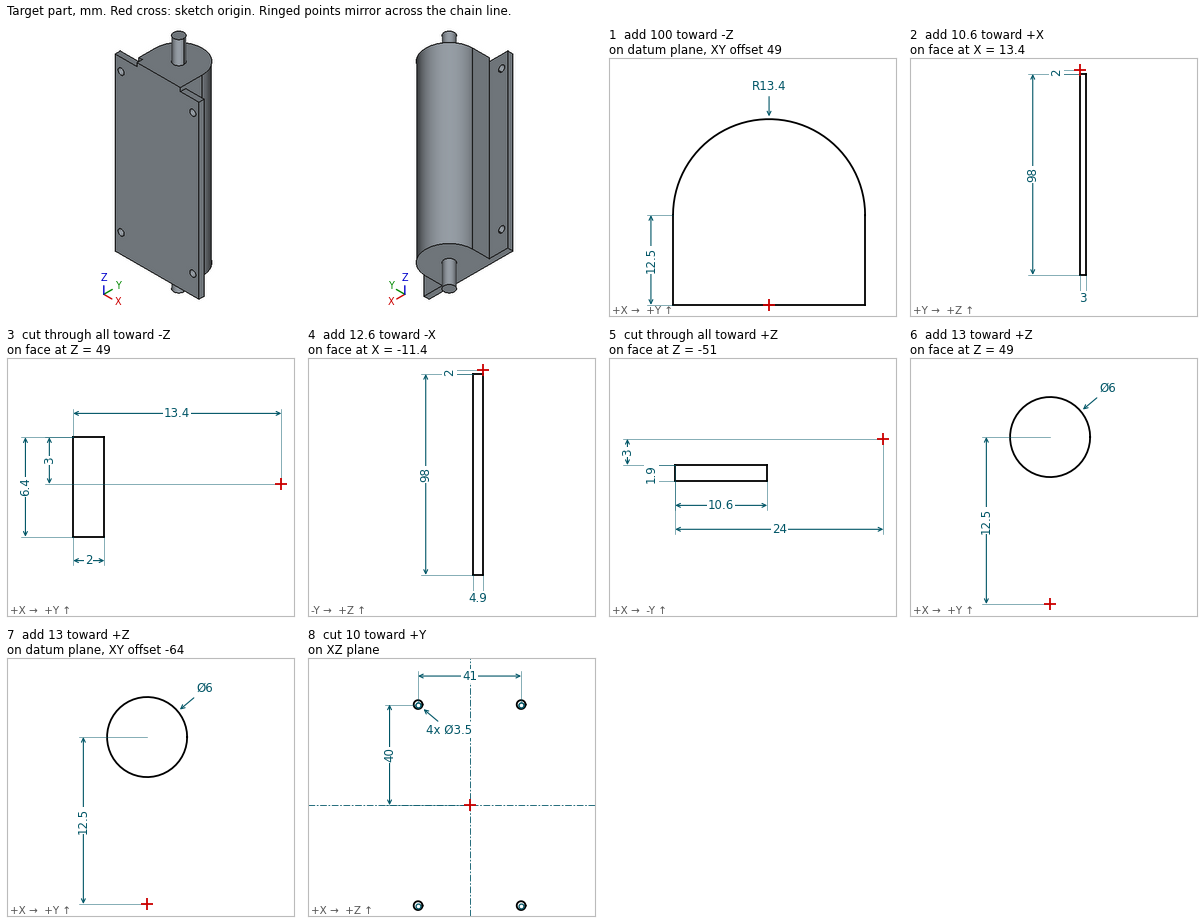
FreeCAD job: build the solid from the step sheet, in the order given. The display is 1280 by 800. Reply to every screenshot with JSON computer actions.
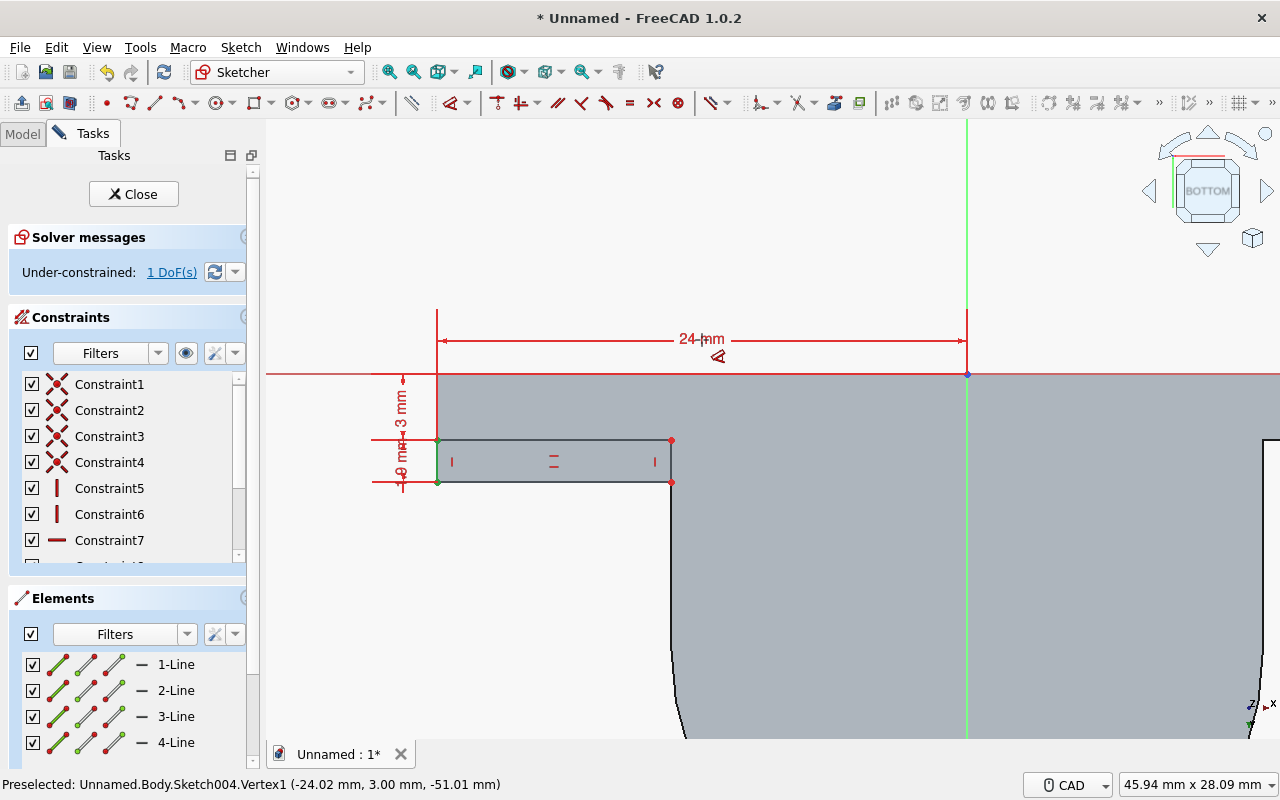
{"action": "left_click", "coordinate": [508, 482]}
{"action": "left_click", "coordinate": [554, 516]}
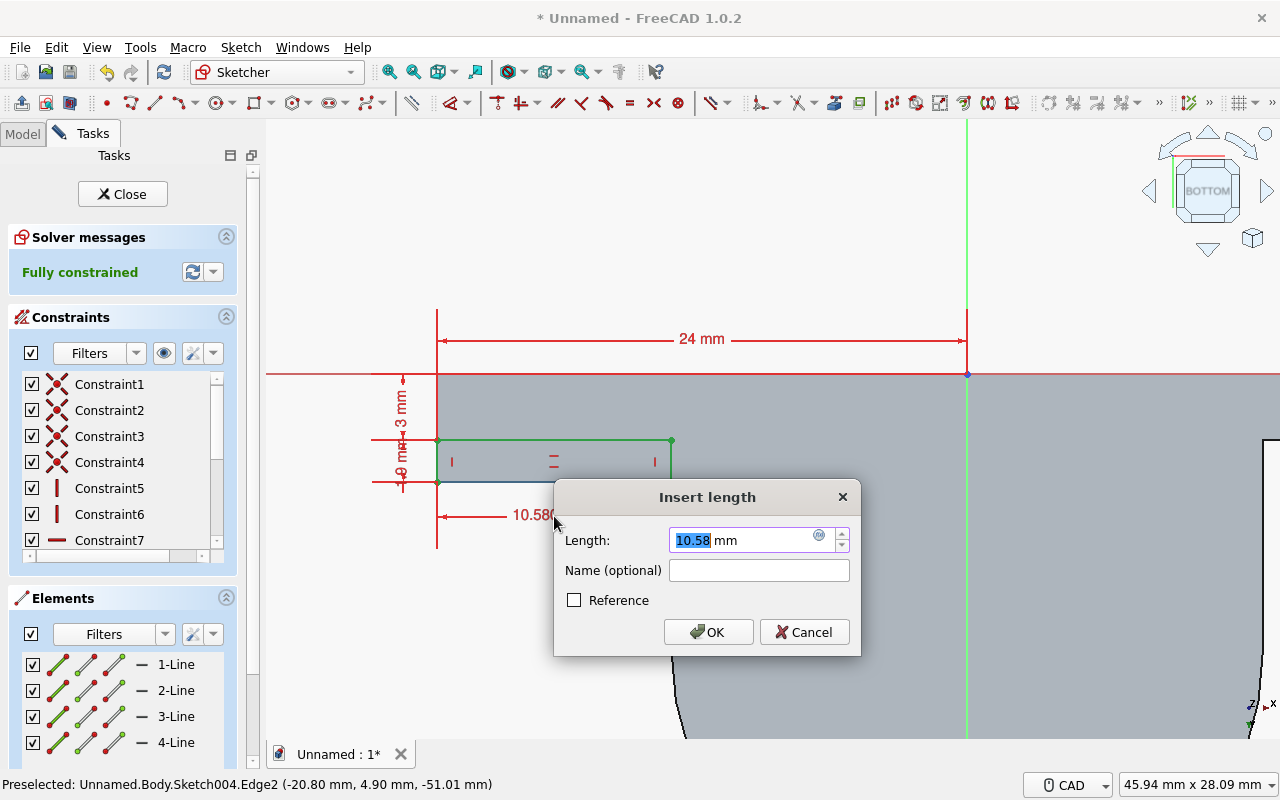
{"action": "type", "text": "10.6"}
{"action": "key", "text": "Return"}
{"action": "key", "text": "Escape"}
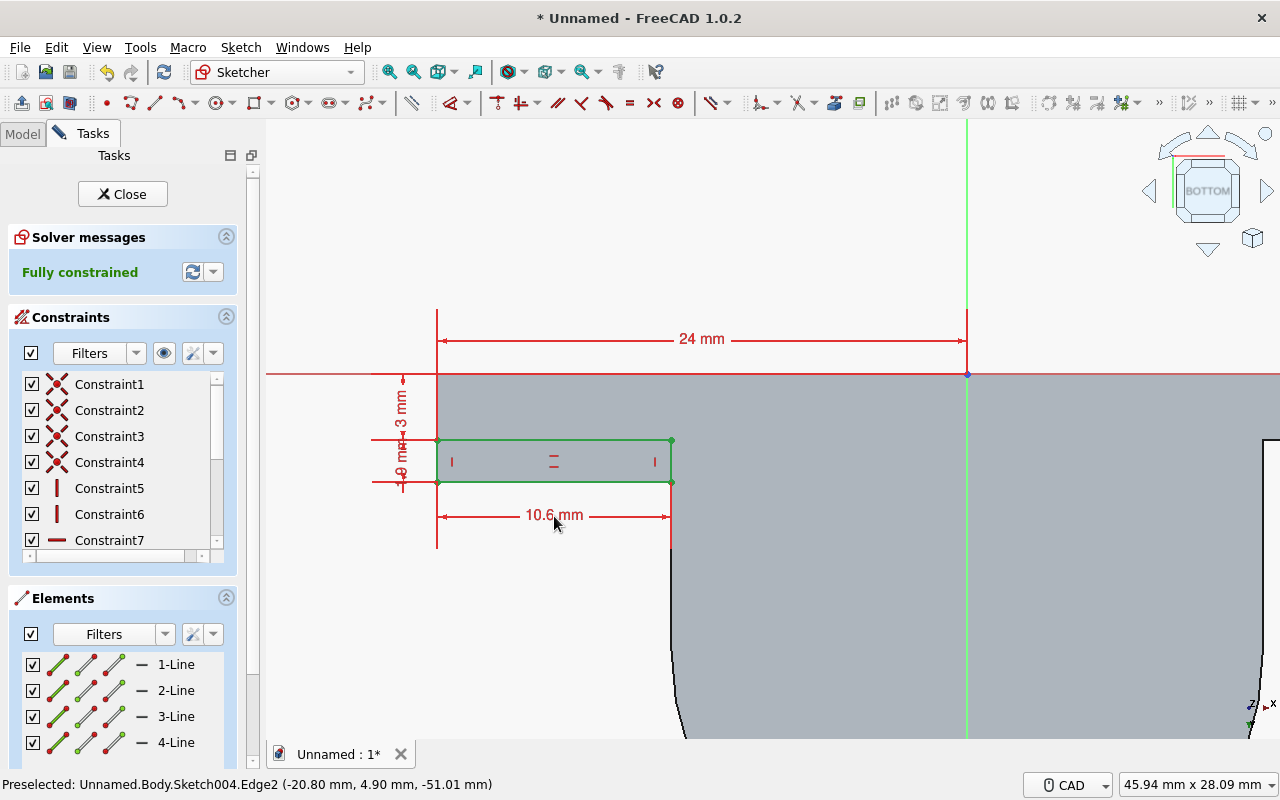
{"action": "left_click", "coordinate": [123, 194]}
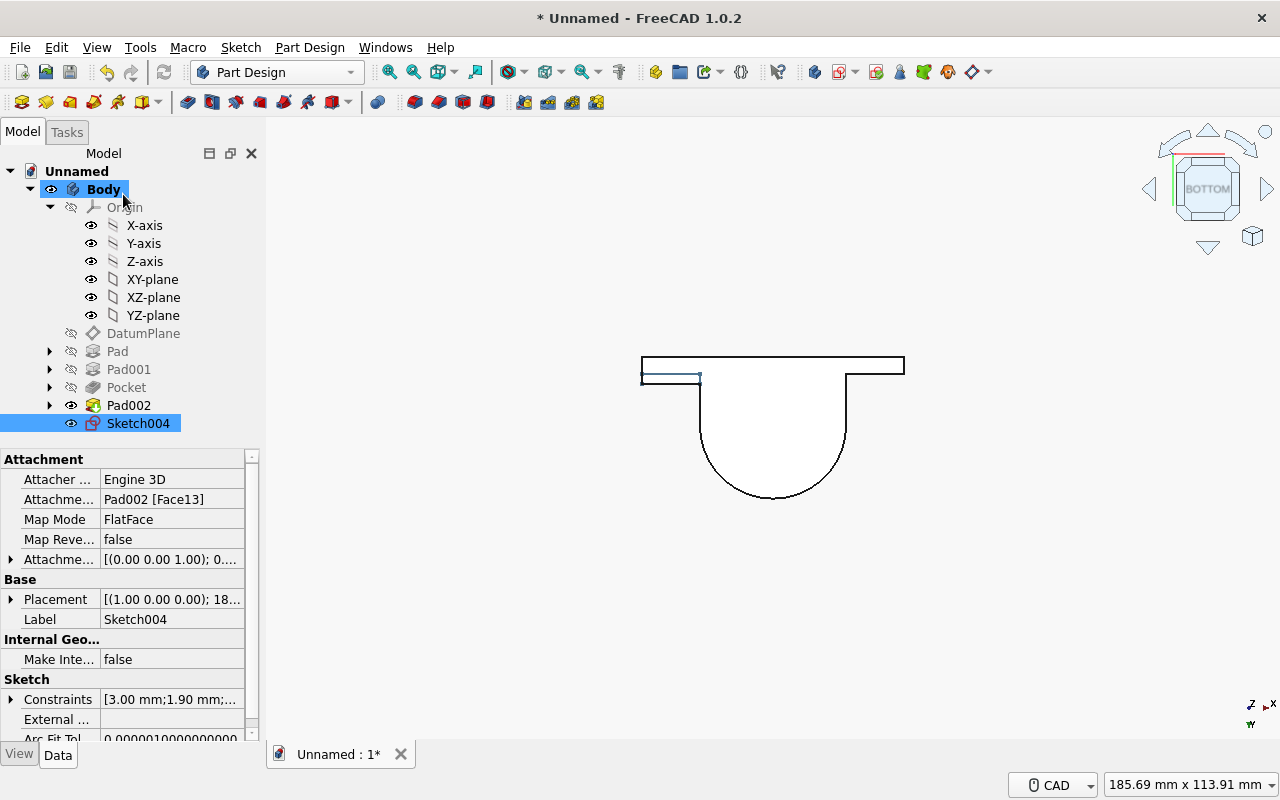
{"action": "left_click", "coordinate": [188, 102]}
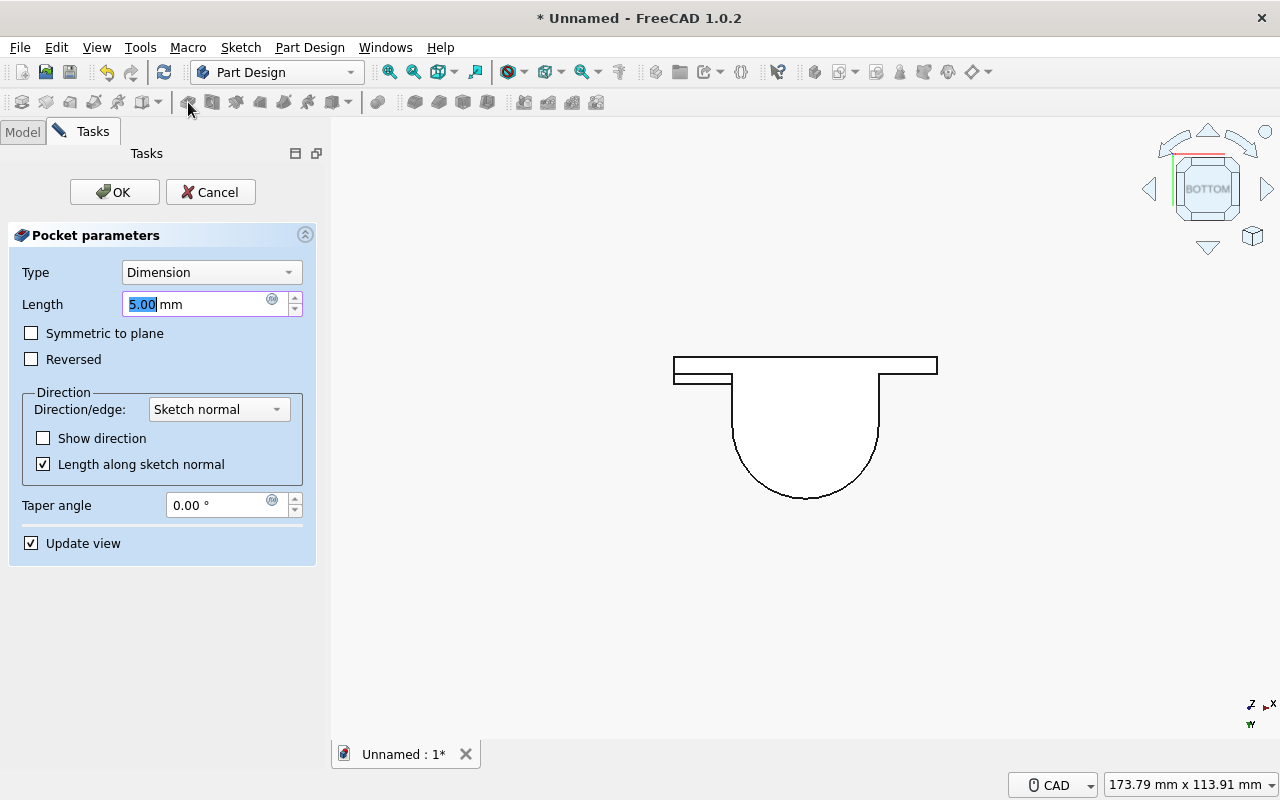
{"action": "left_click", "coordinate": [212, 272]}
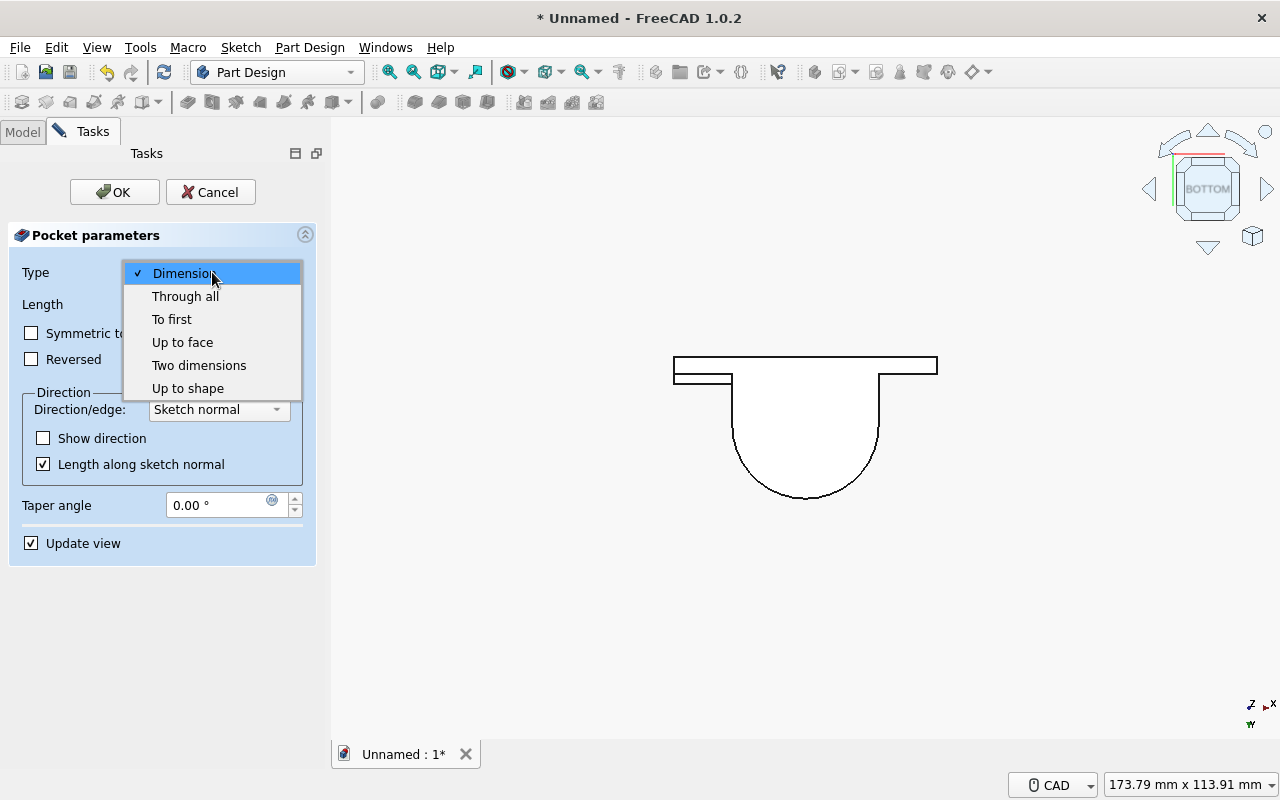
{"action": "left_click", "coordinate": [212, 296]}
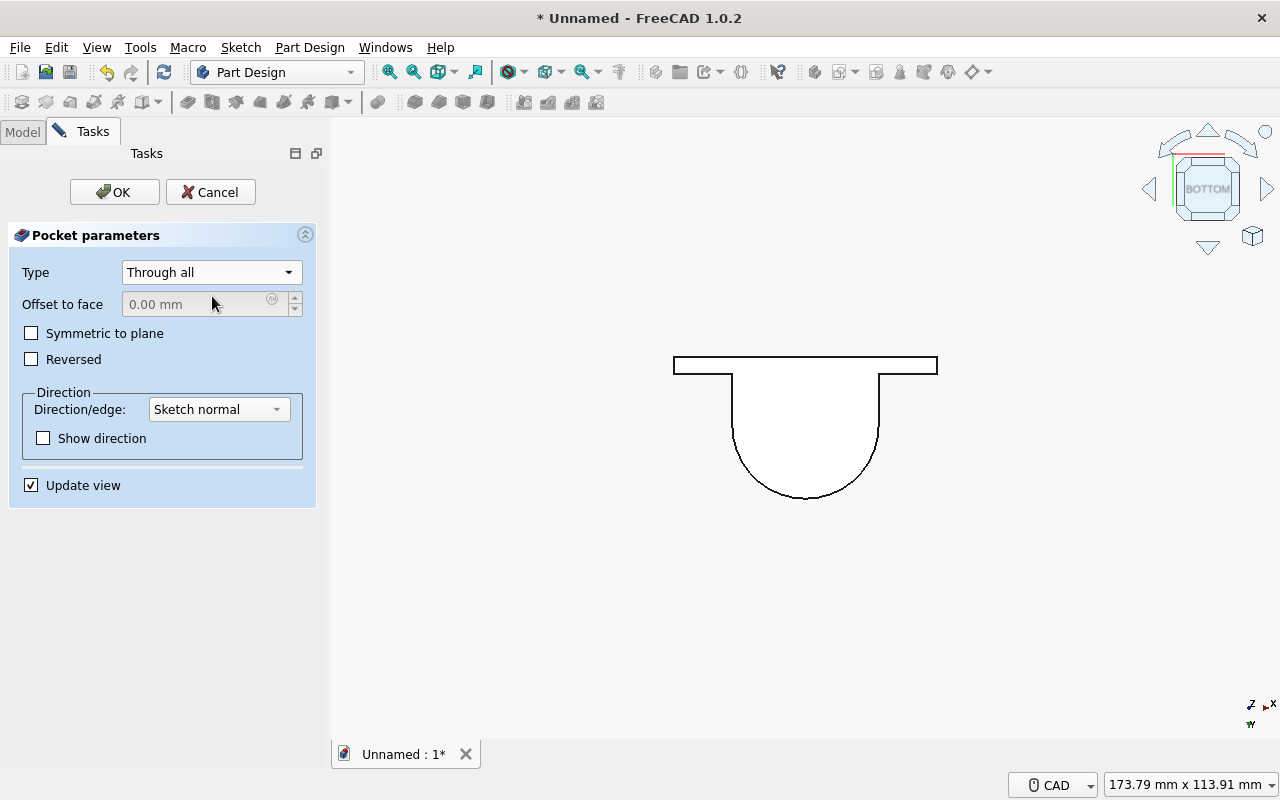
{"action": "left_click", "coordinate": [115, 192]}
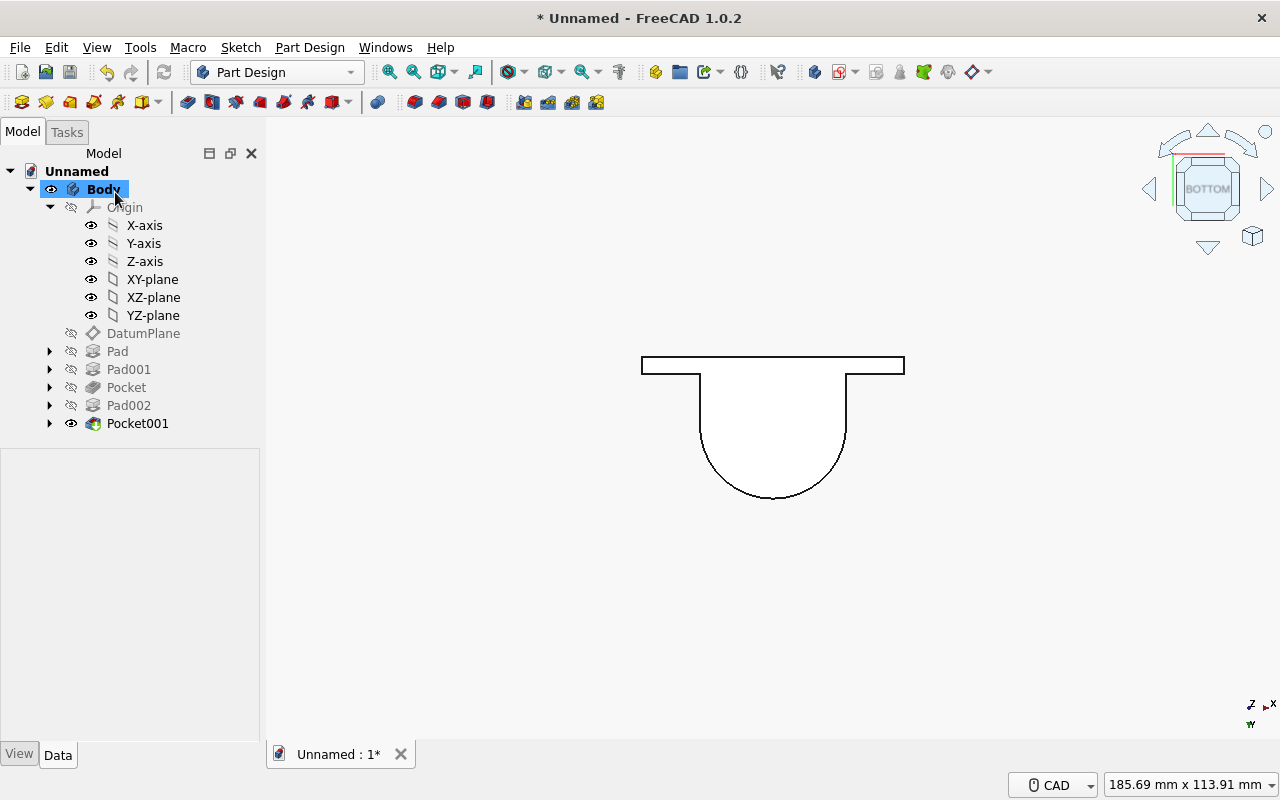
{"action": "left_click", "coordinate": [390, 72]}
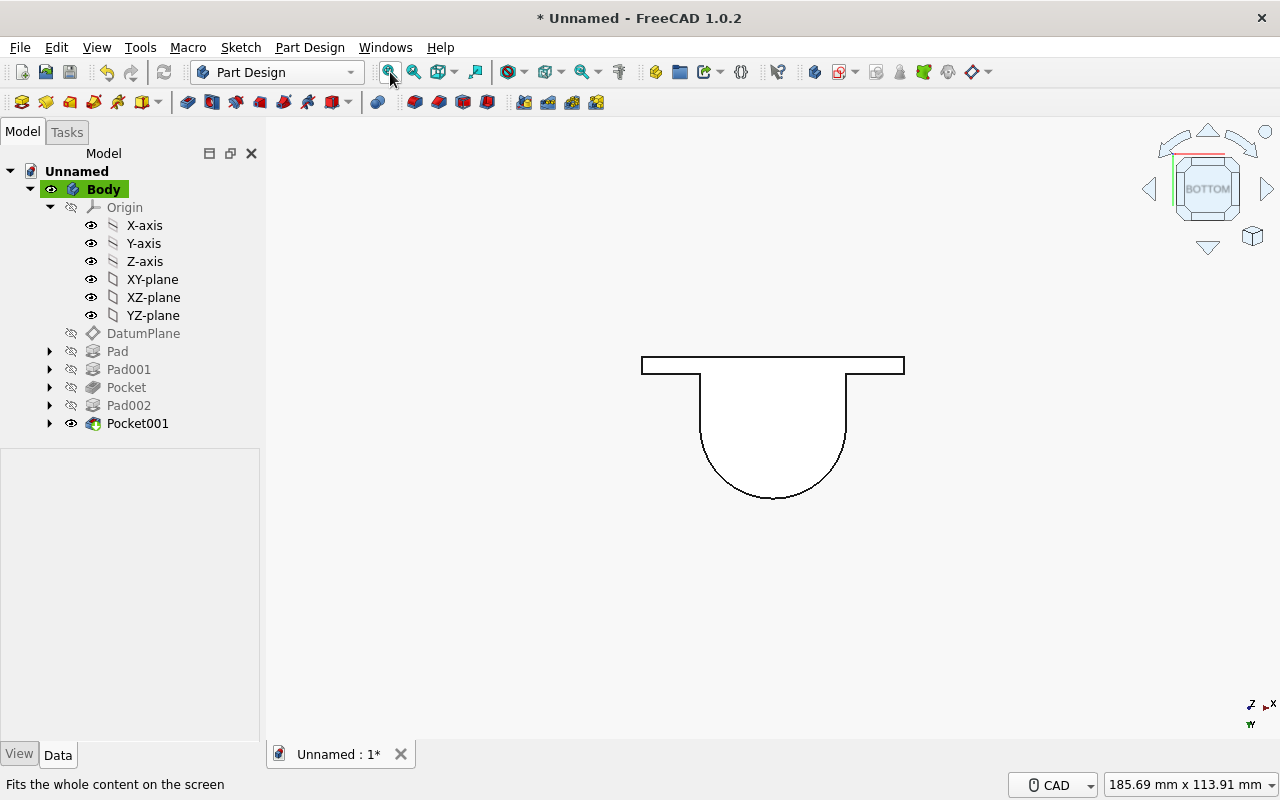
{"action": "key", "text": "0"}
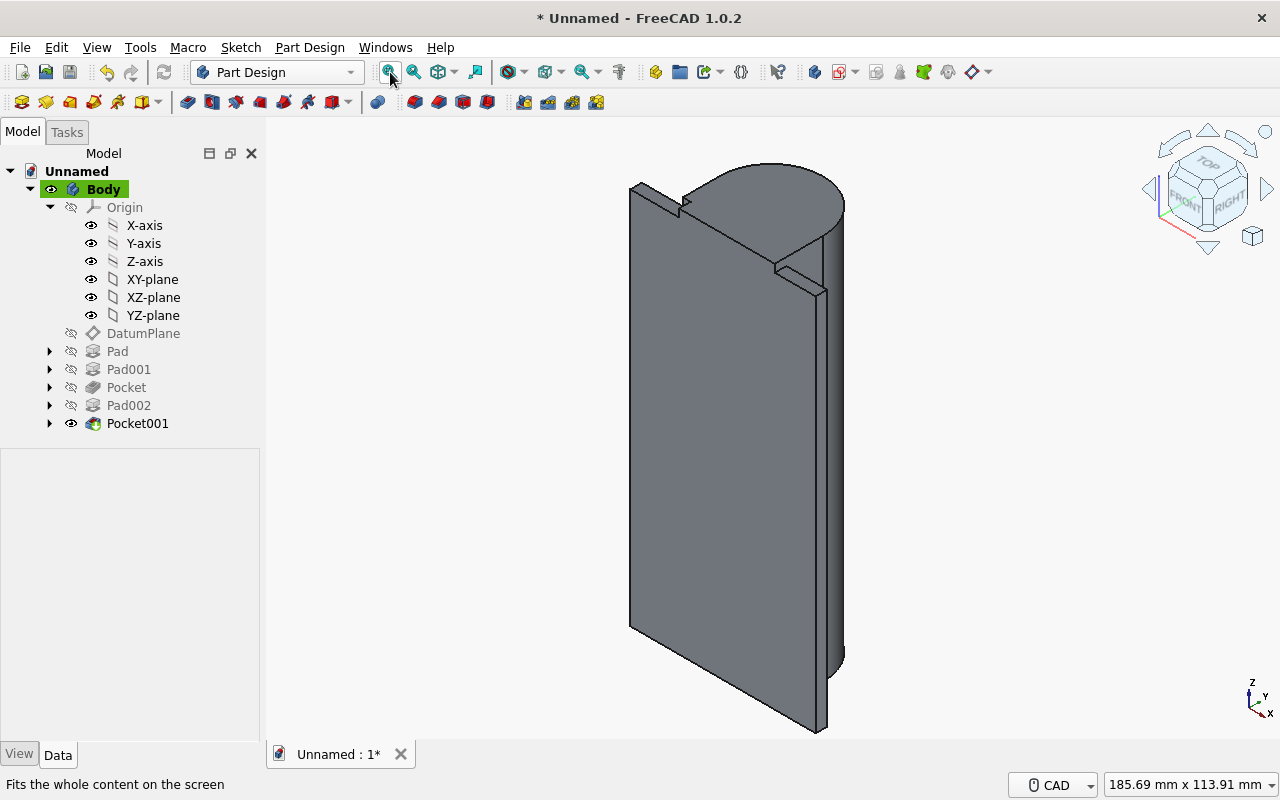
{"action": "left_click", "coordinate": [773, 204]}